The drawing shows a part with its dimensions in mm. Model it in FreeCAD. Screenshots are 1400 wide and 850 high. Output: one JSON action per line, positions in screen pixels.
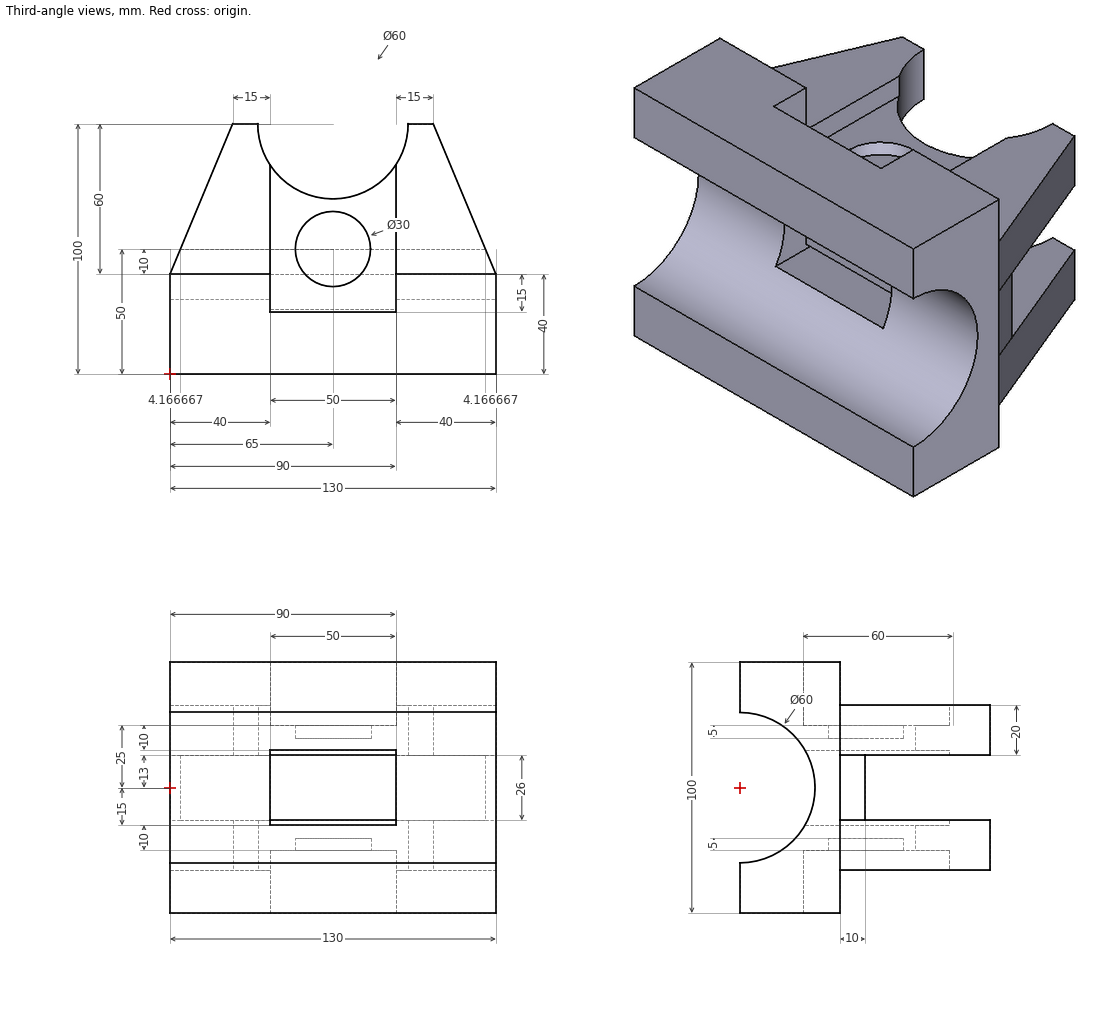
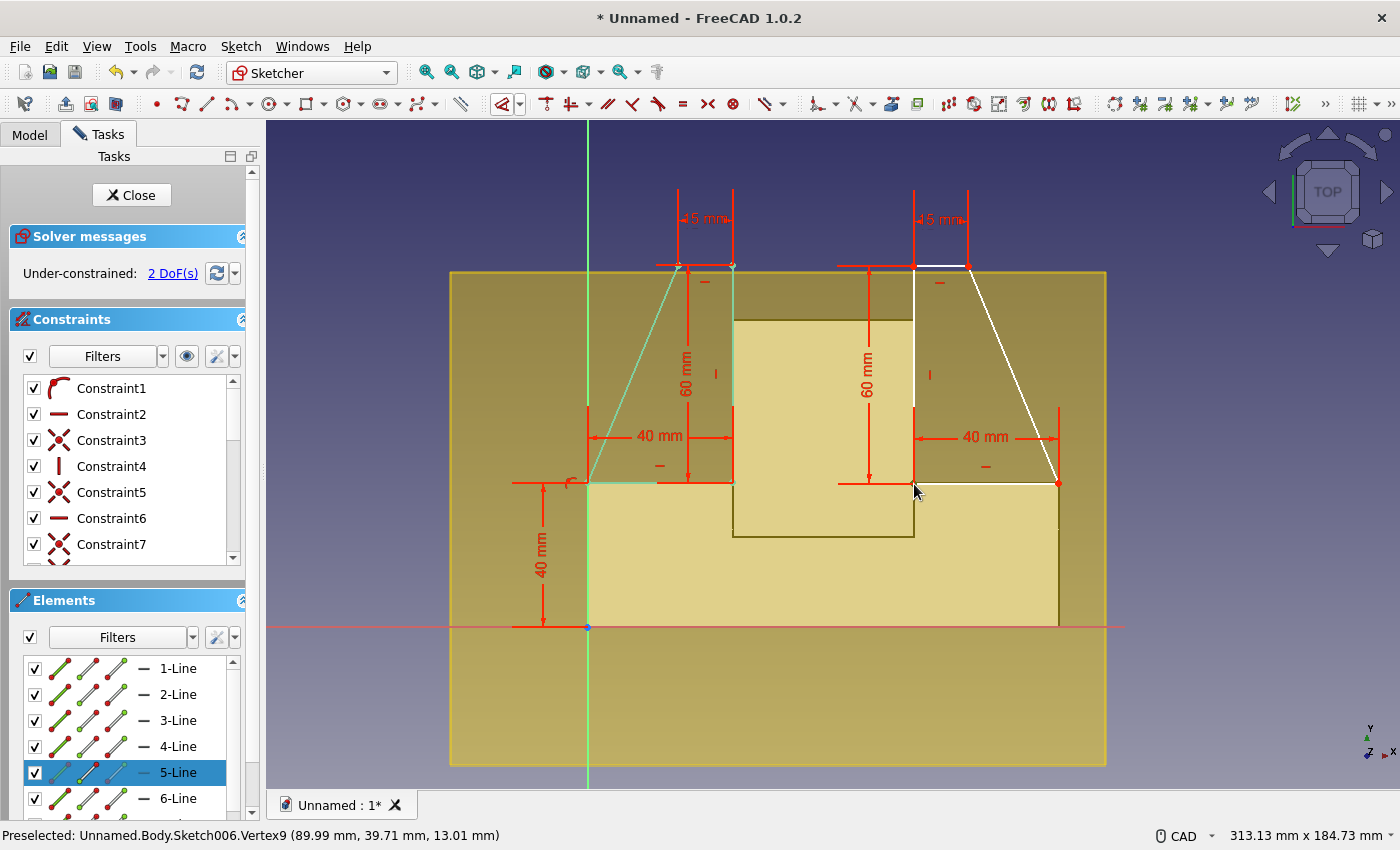
{"action": "key", "text": "l"}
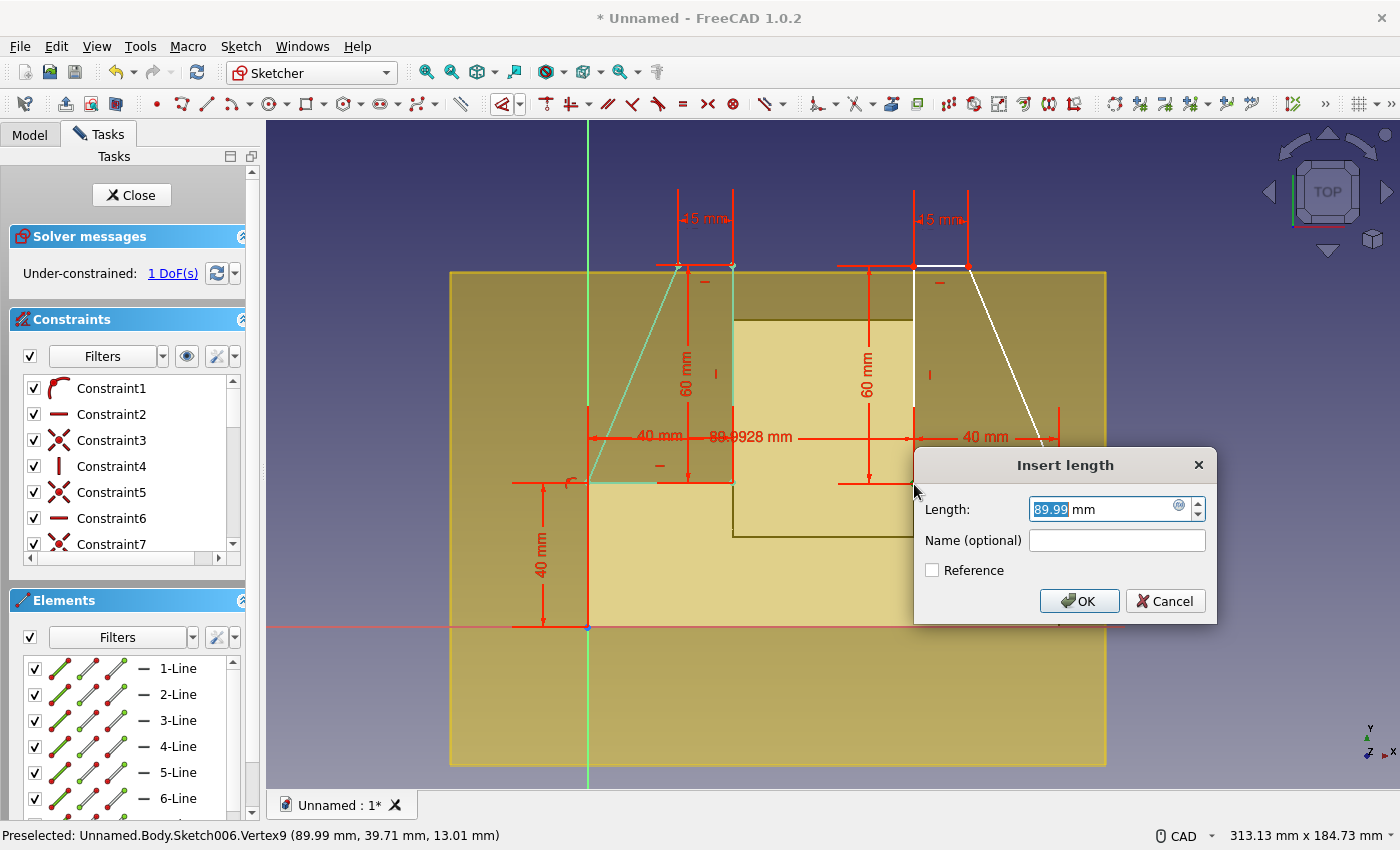
{"action": "type", "text": "90"}
{"action": "key", "text": "Return"}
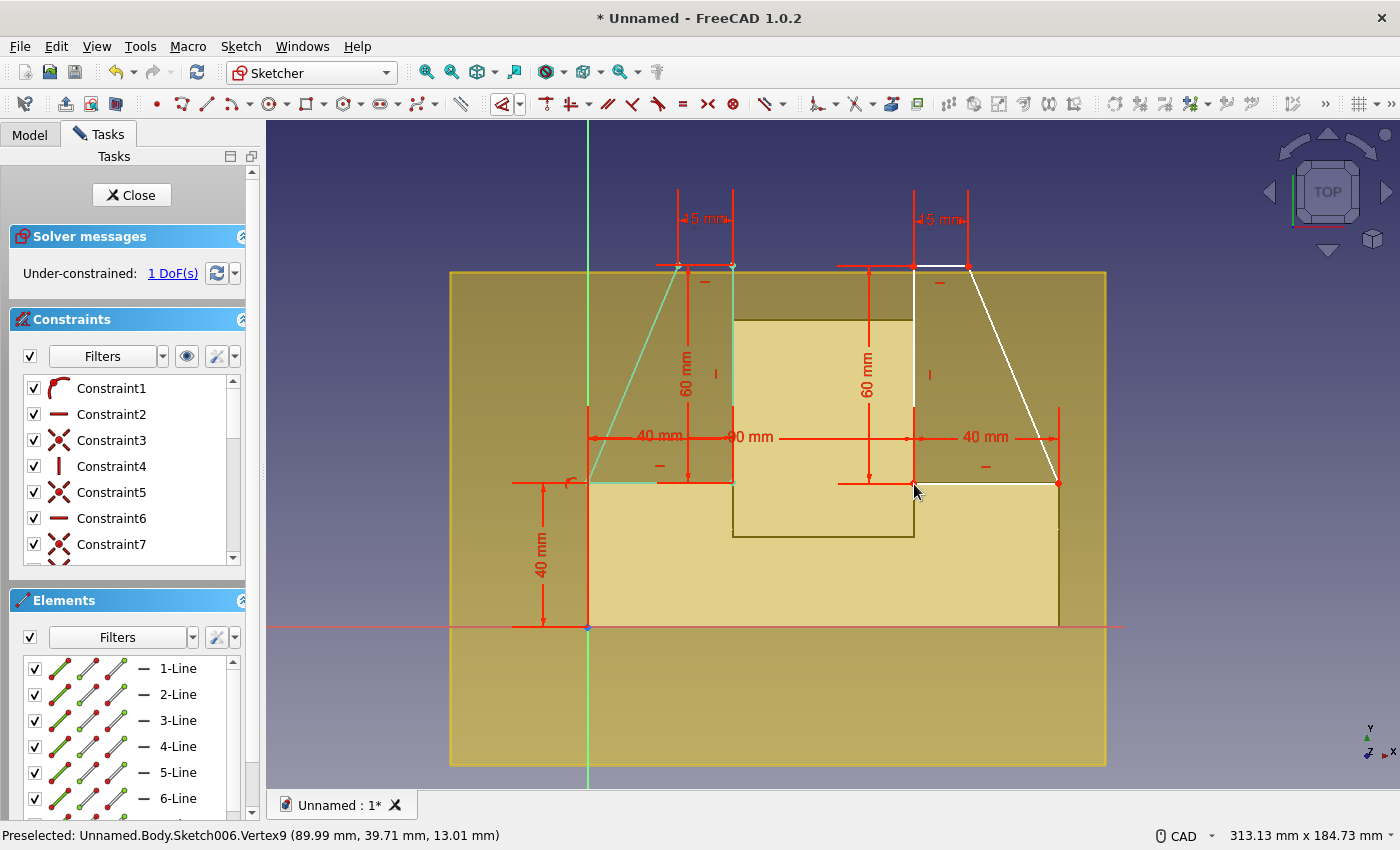
{"action": "left_click", "coordinate": [914, 484]}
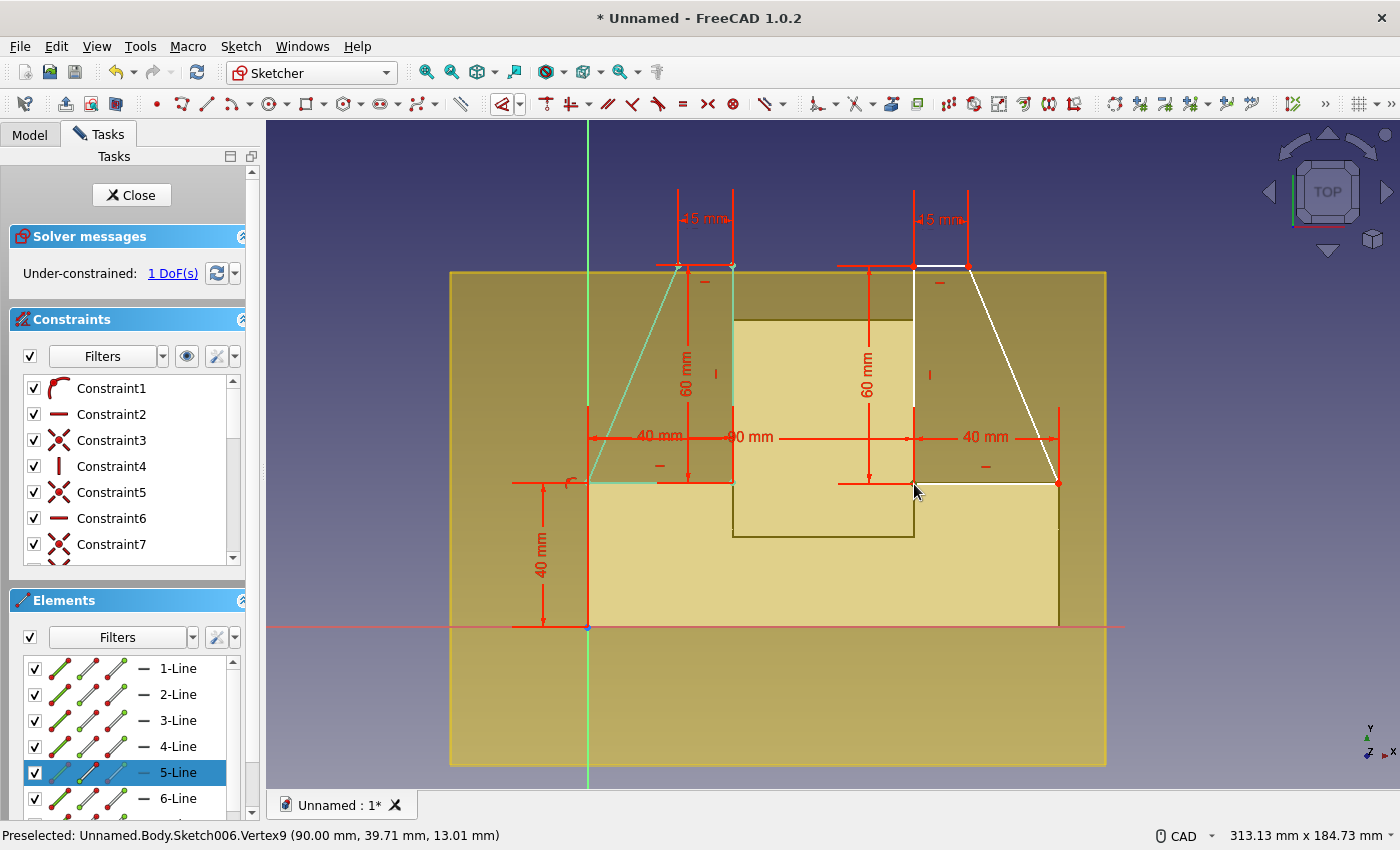
{"action": "left_click", "coordinate": [520, 104]}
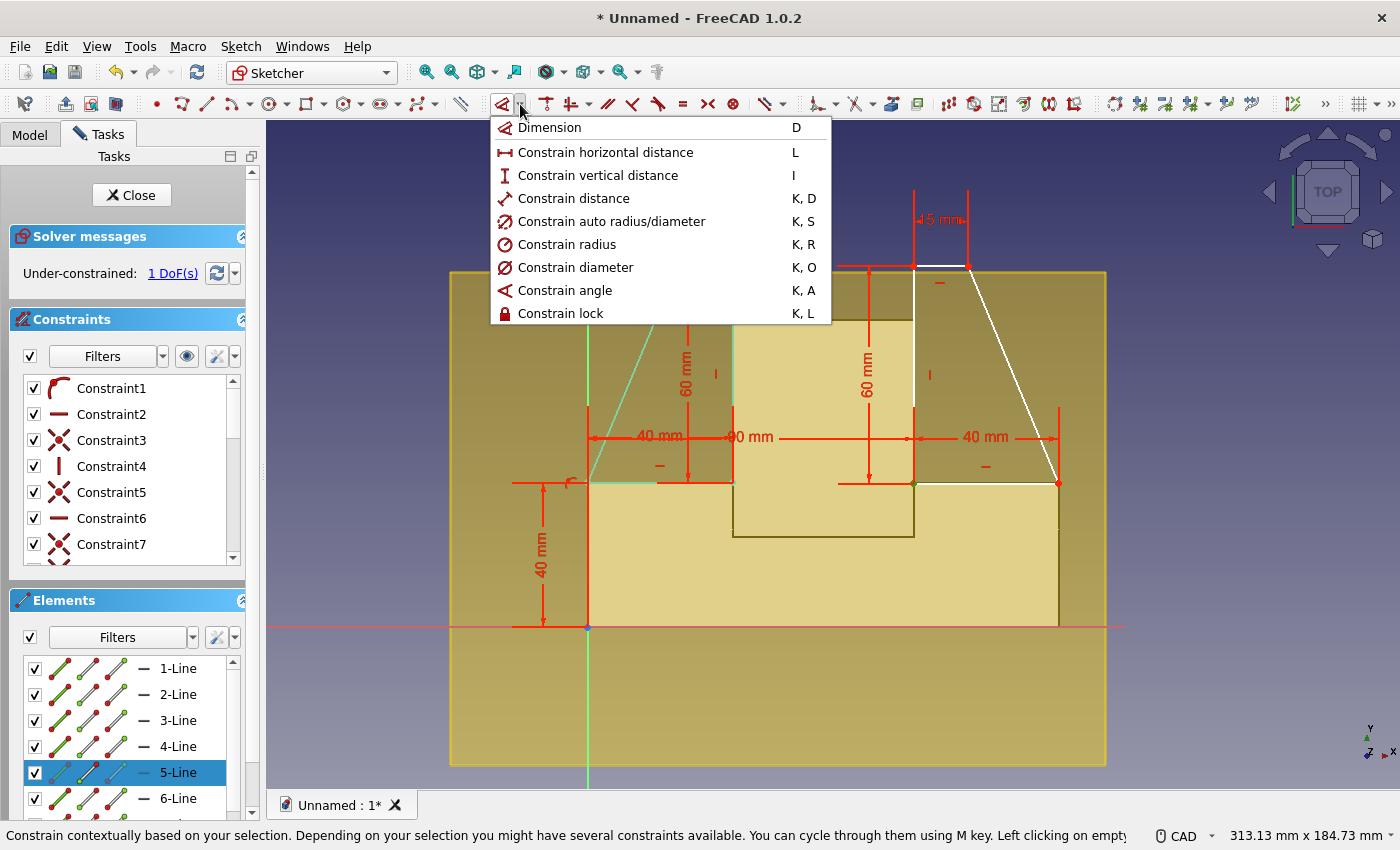
{"action": "left_click", "coordinate": [661, 176]}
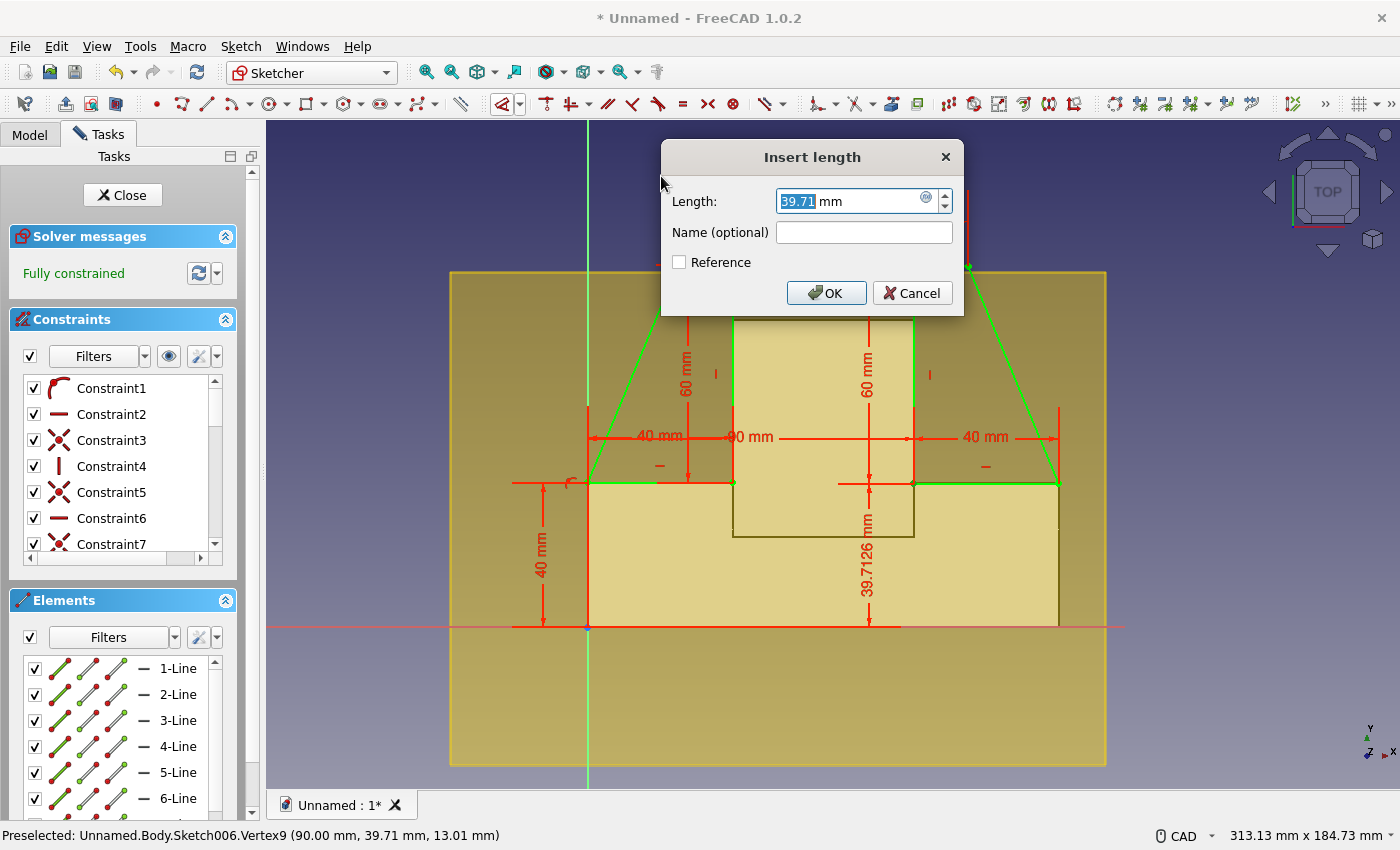
{"action": "type", "text": "40"}
{"action": "key", "text": "Return"}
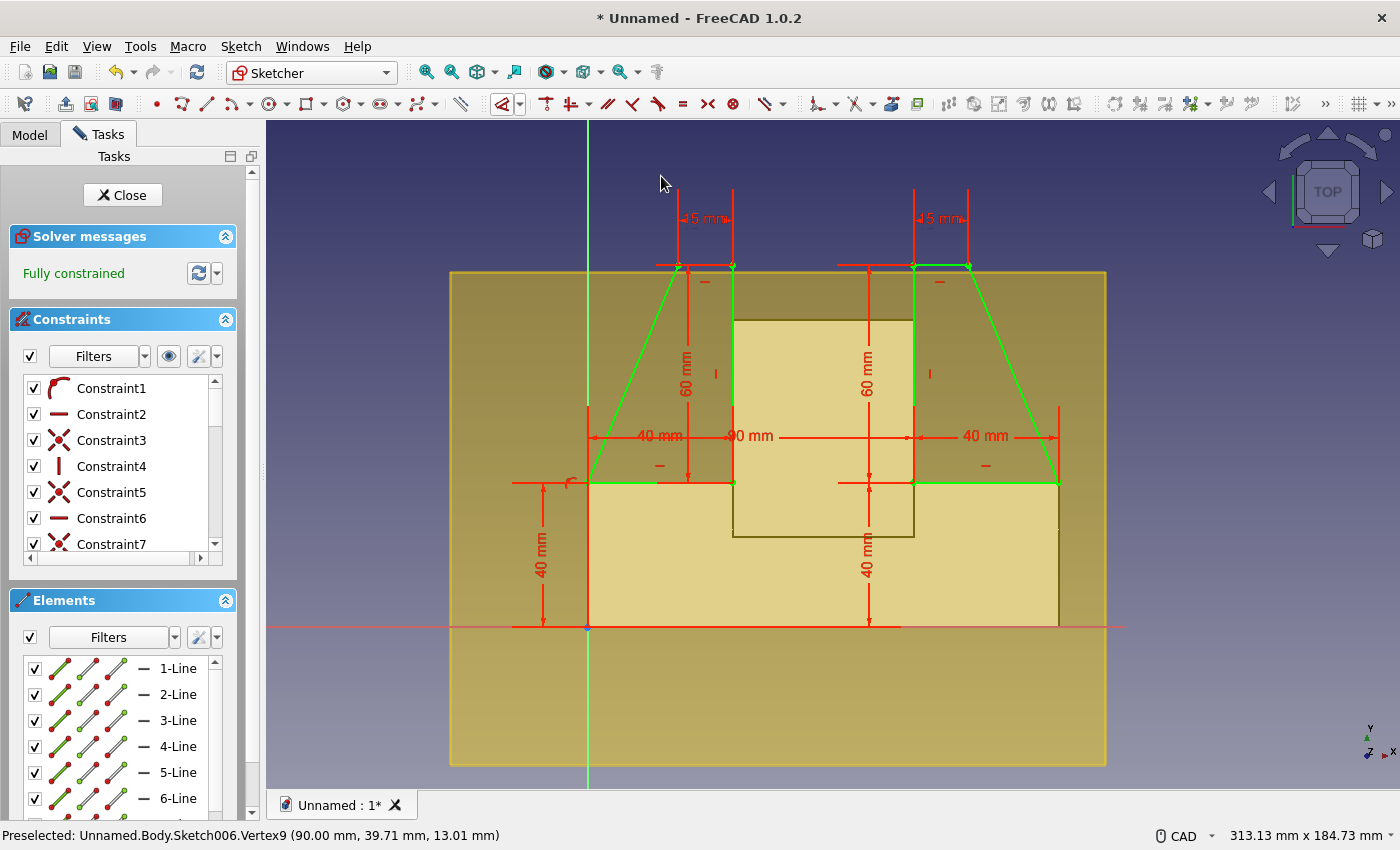
{"action": "left_click", "coordinate": [123, 195]}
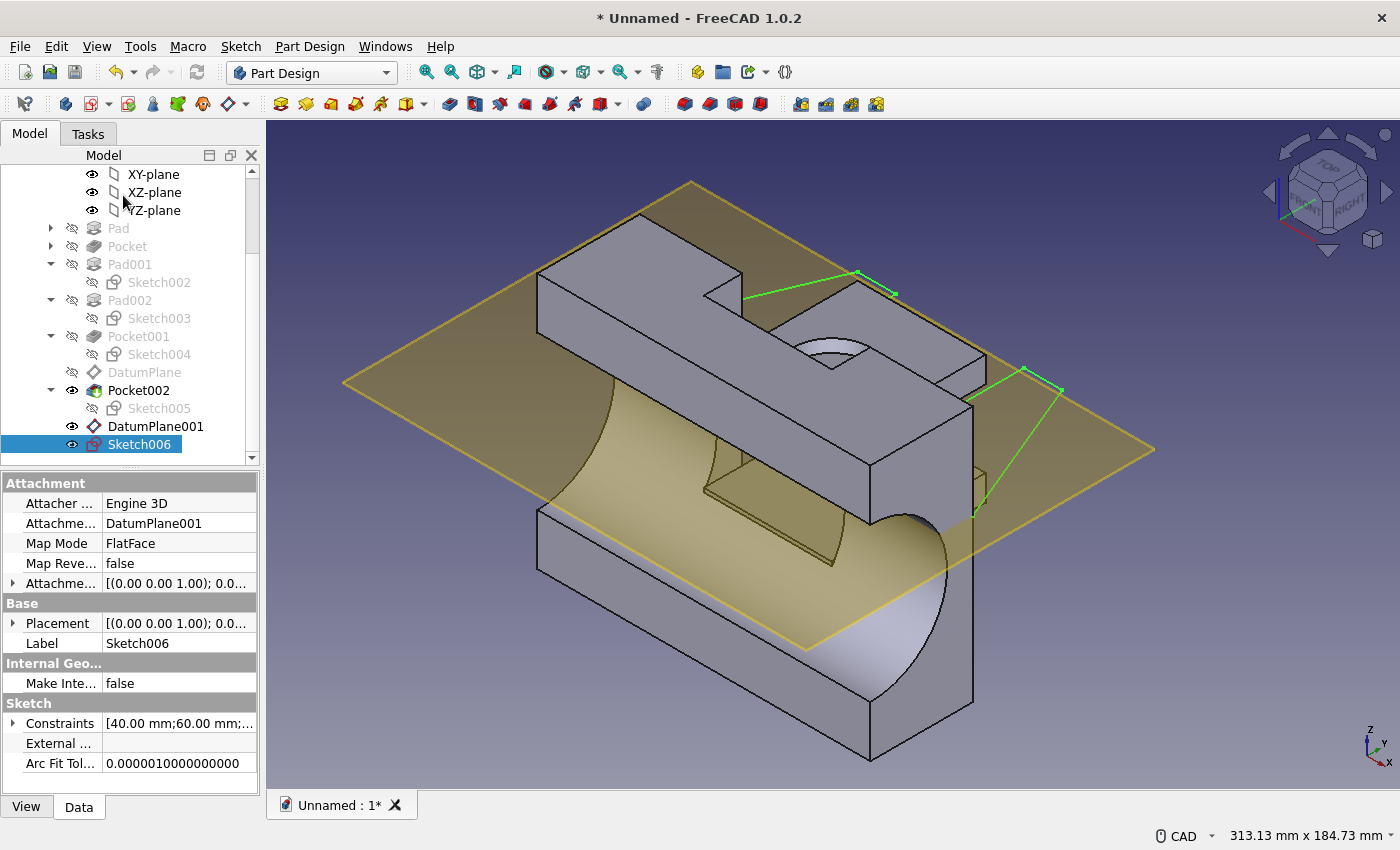
{"action": "left_click", "coordinate": [281, 104]}